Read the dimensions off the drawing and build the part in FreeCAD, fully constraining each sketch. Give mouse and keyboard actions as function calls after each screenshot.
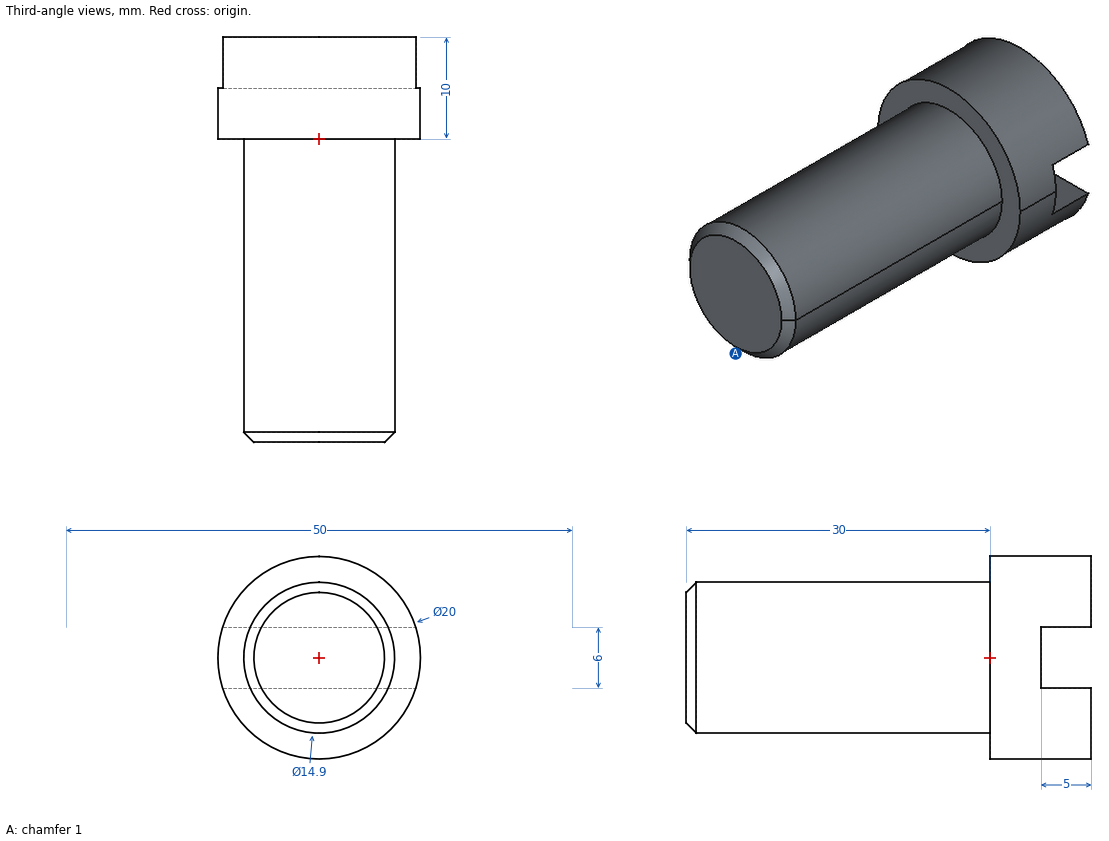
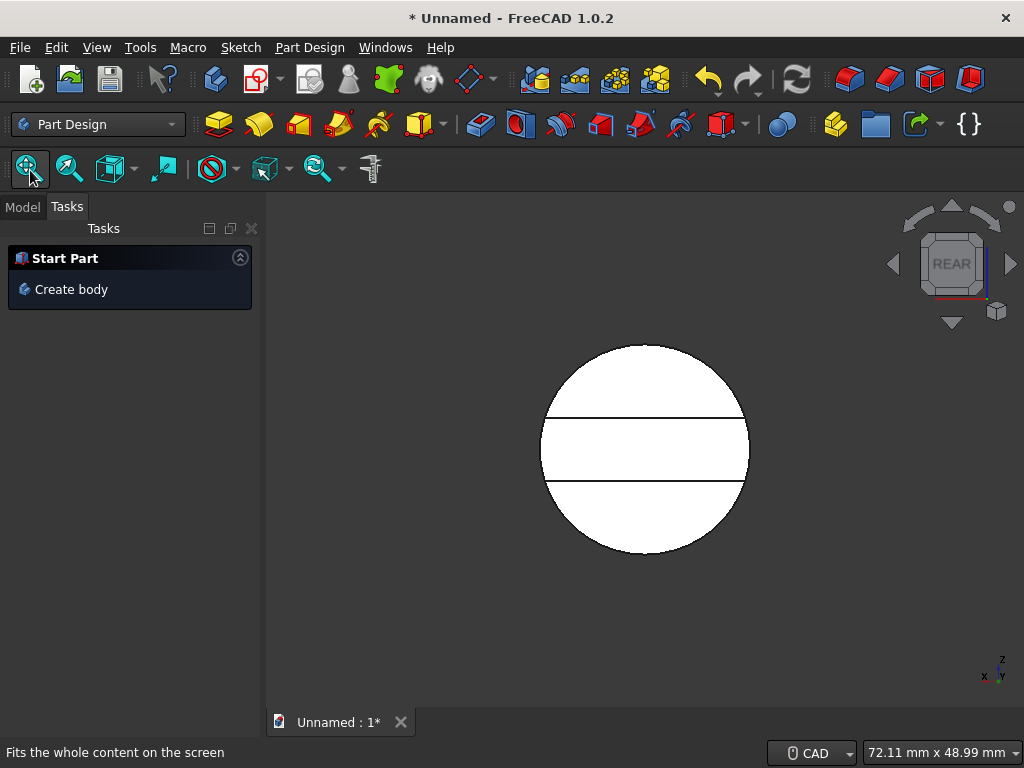
key(0)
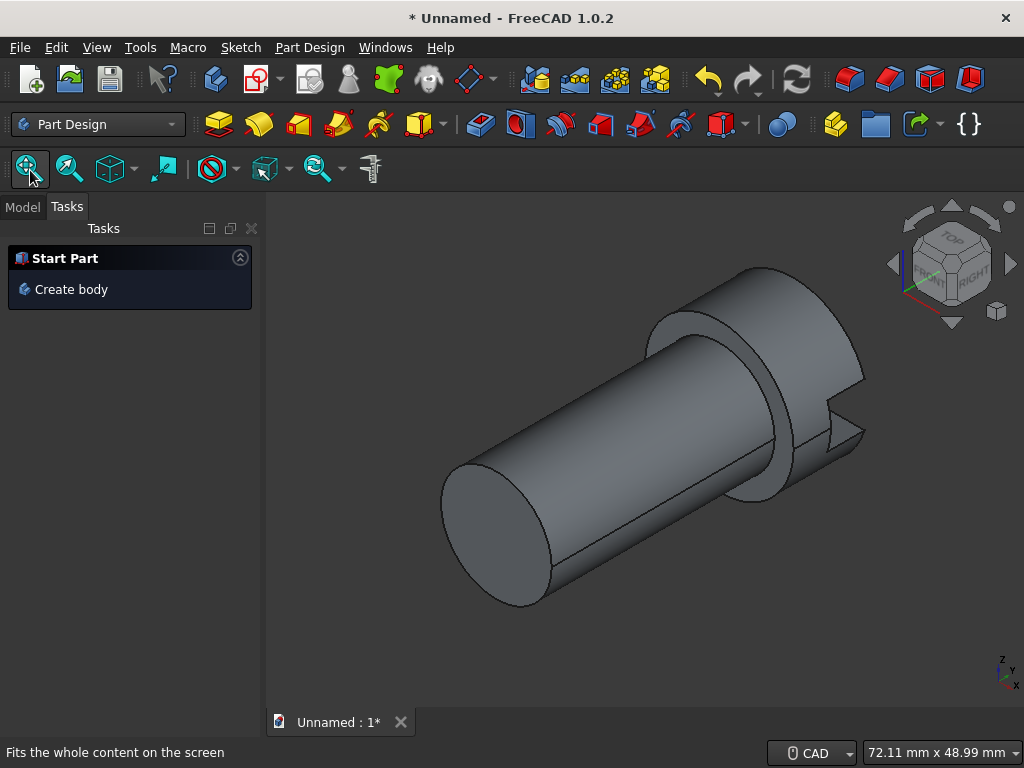
click(479, 464)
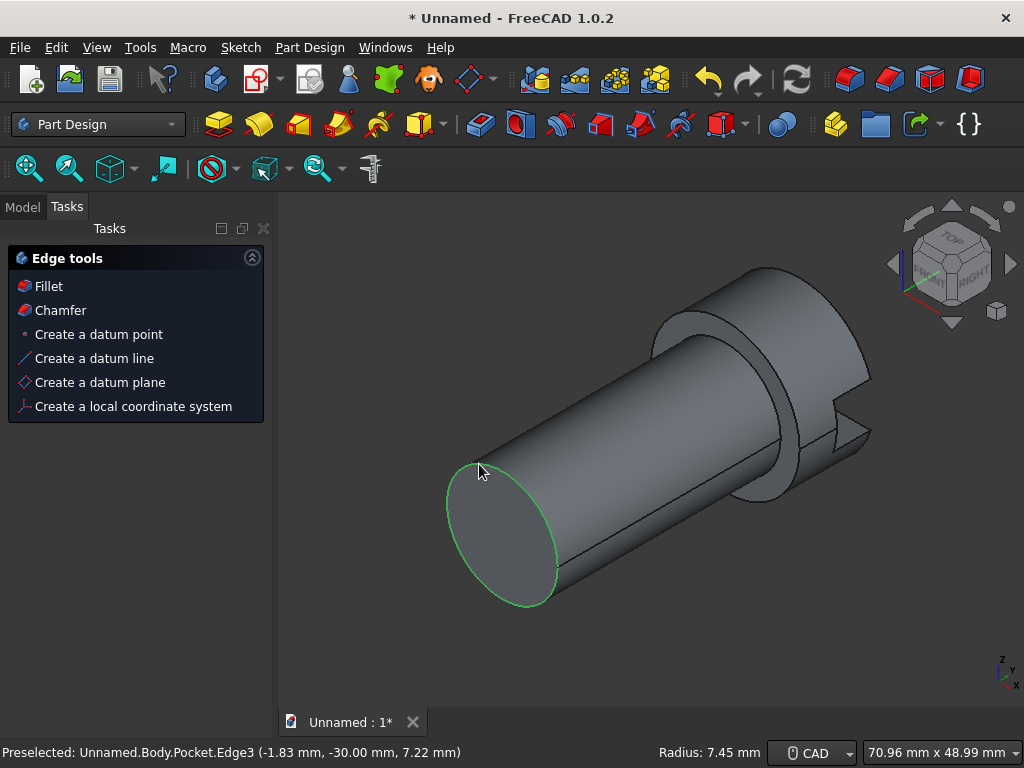
click(890, 80)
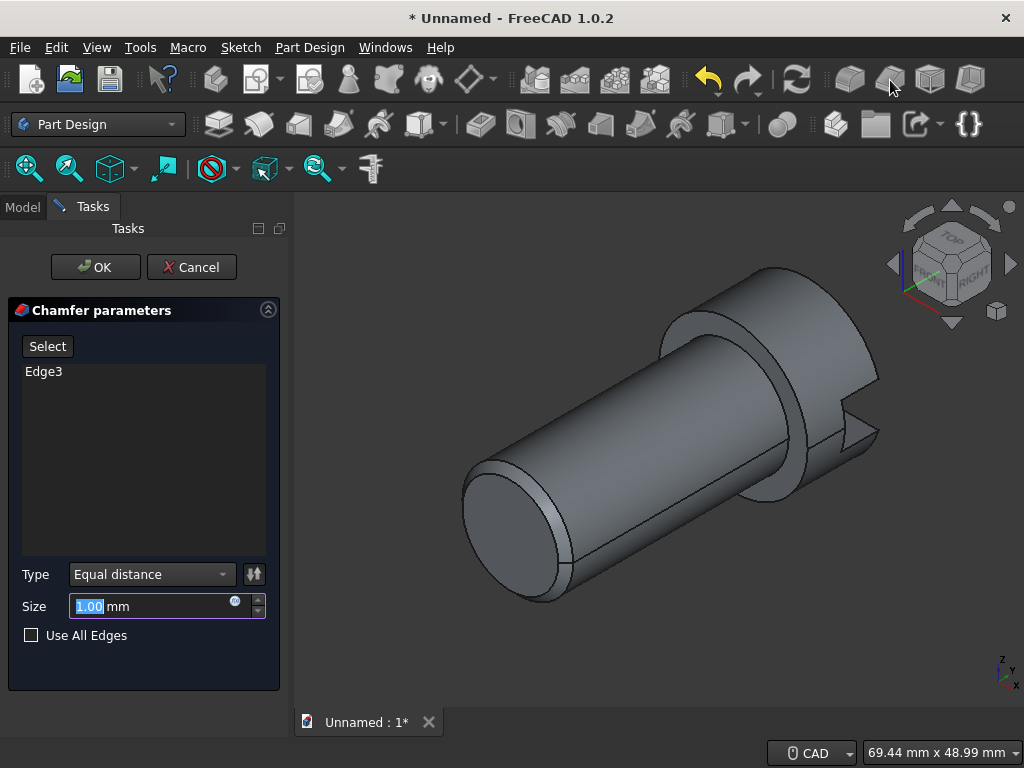
text(1)
key(Tab)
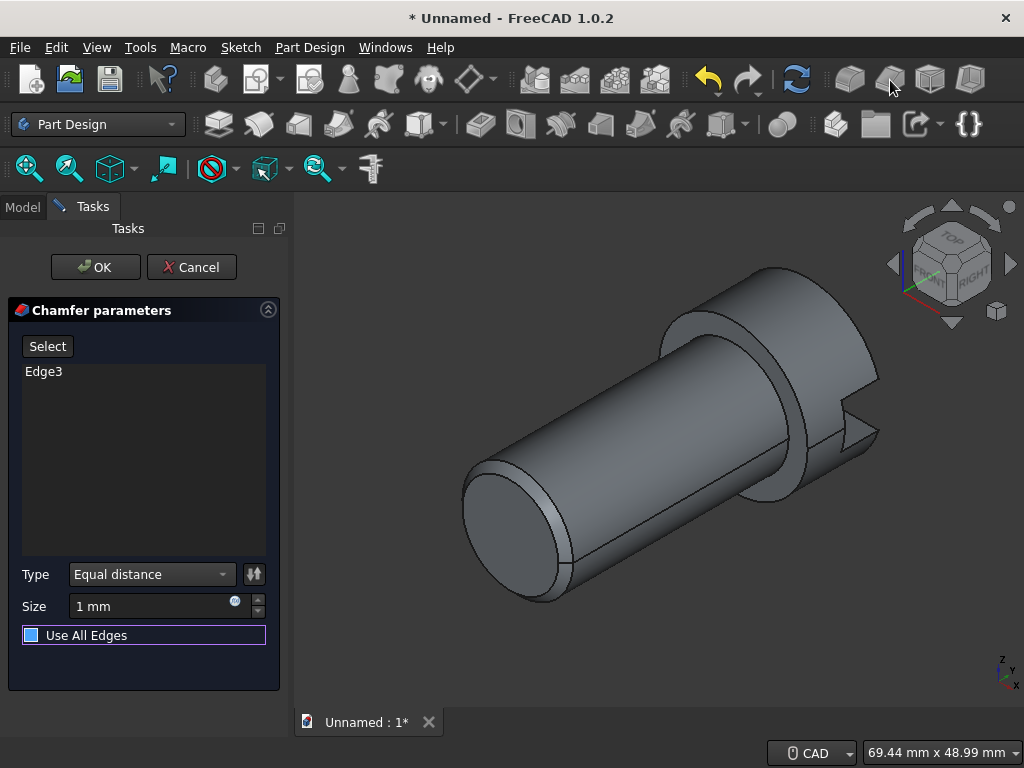
click(96, 267)